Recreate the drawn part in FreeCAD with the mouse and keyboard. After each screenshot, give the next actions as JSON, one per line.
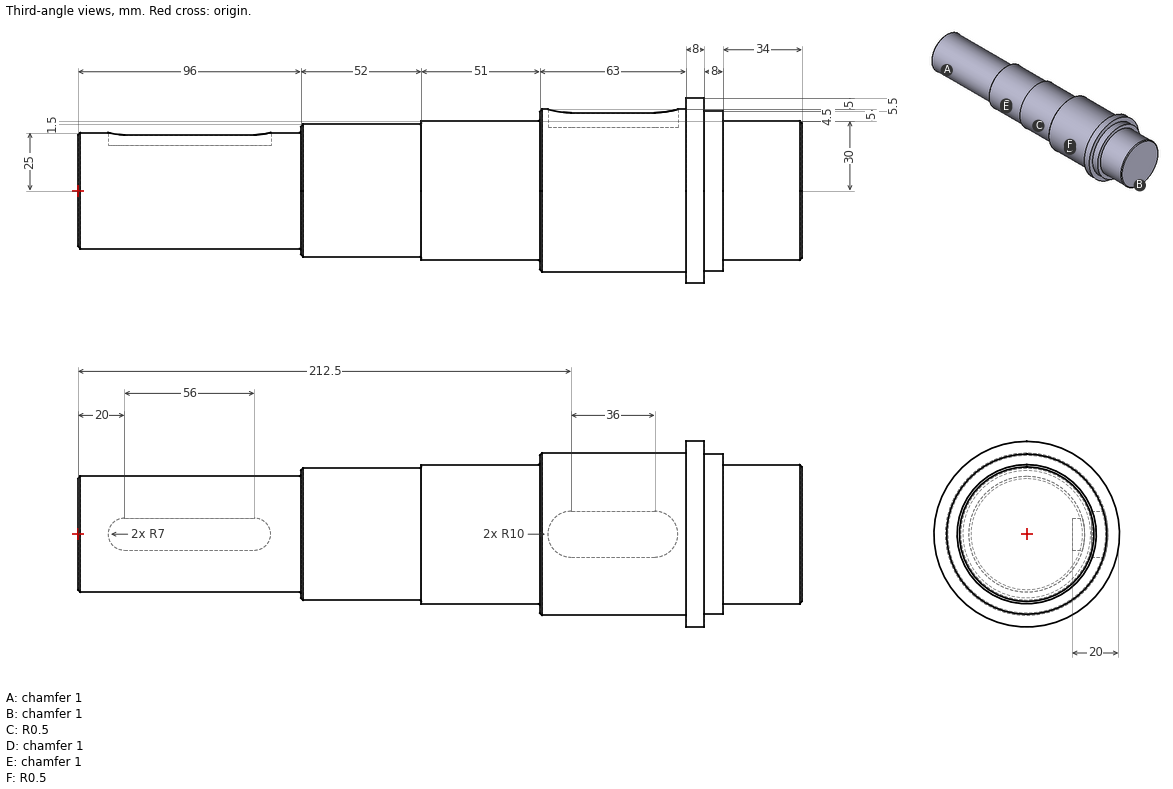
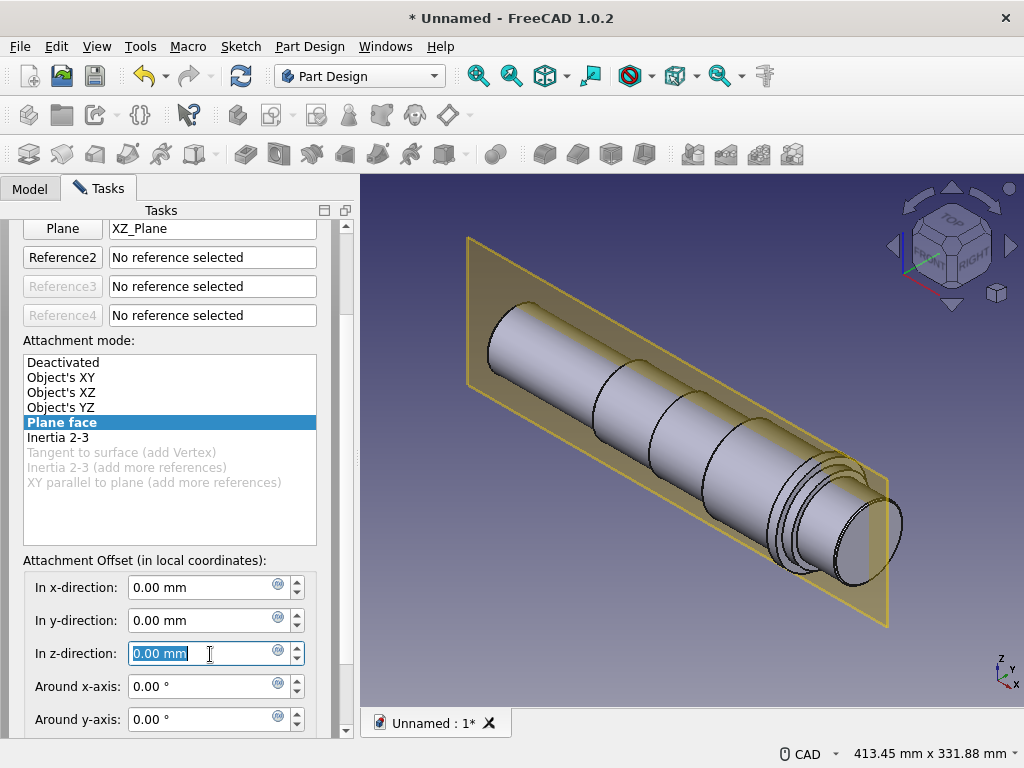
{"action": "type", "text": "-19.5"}
{"action": "key", "text": "Tab"}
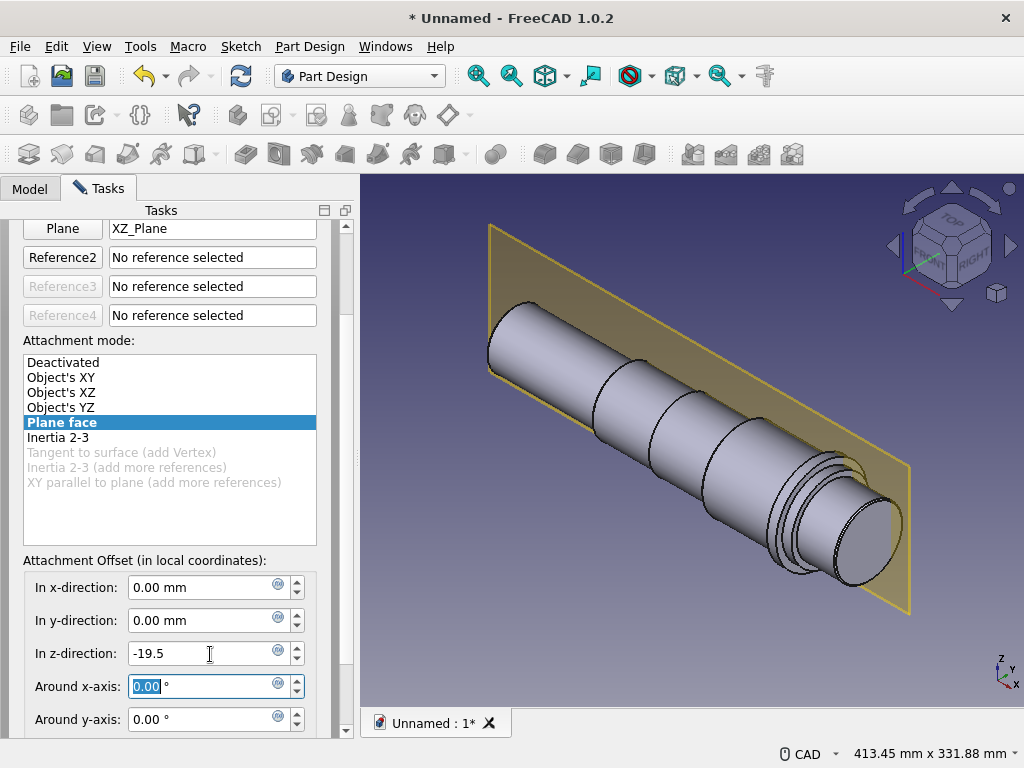
{"action": "scroll", "coordinate": [346, 479], "scroll_direction": "up", "scroll_amount": 3}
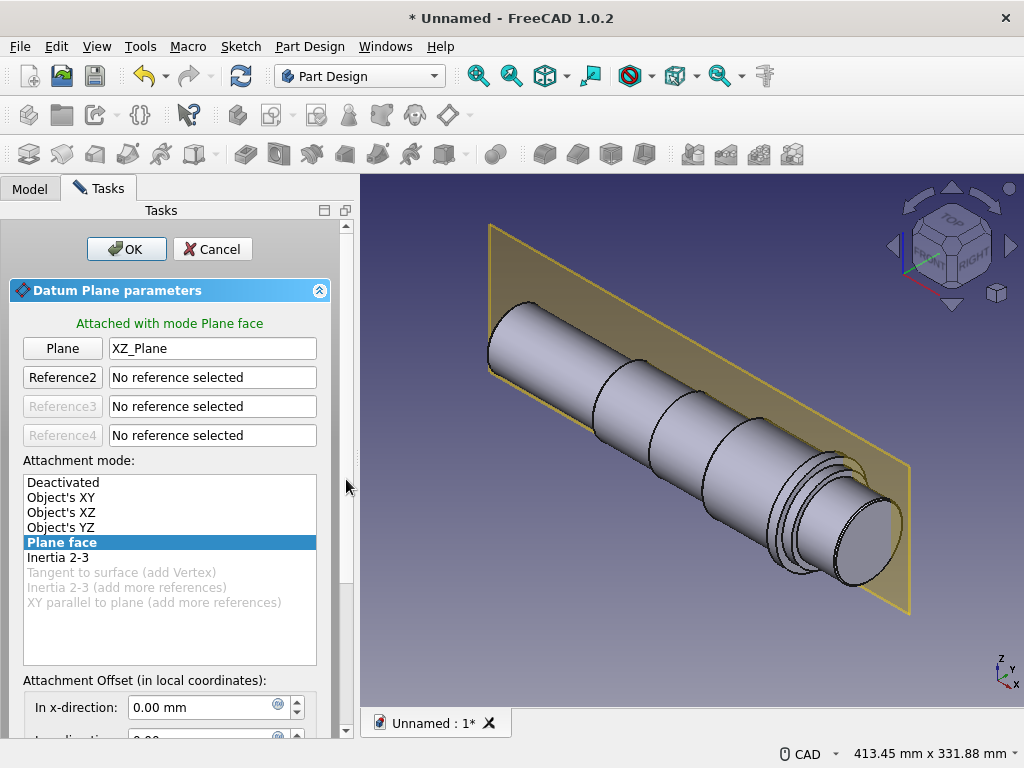
{"action": "left_click", "coordinate": [127, 249]}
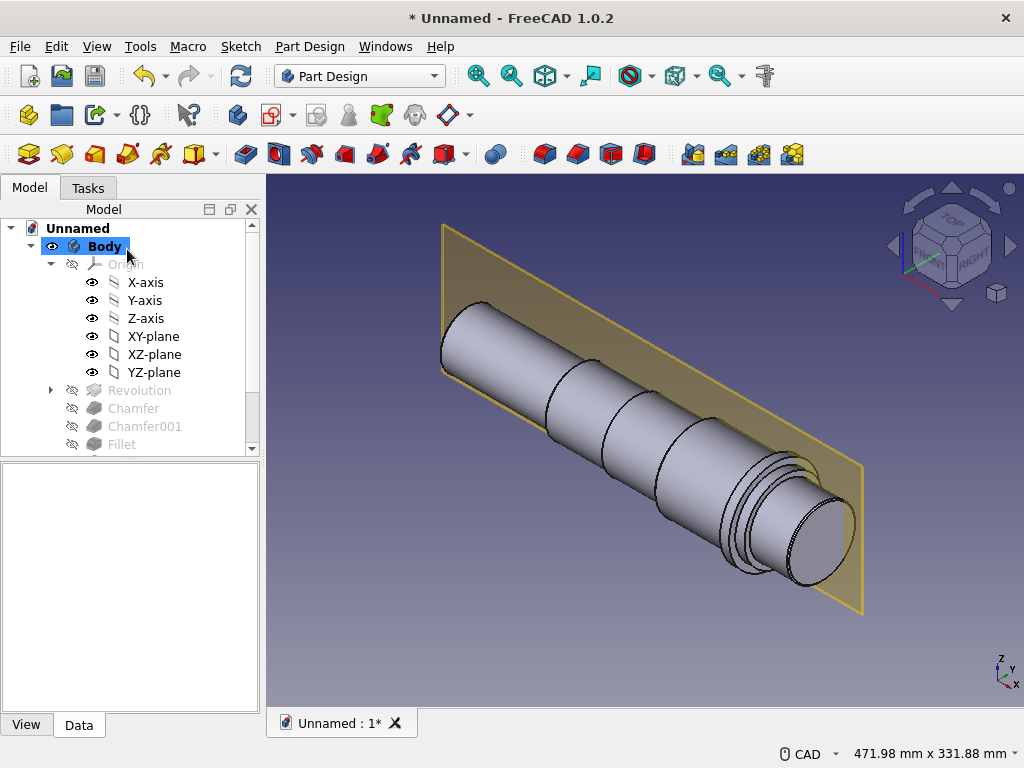
{"action": "scroll", "coordinate": [101, 332], "scroll_direction": "down", "scroll_amount": 3}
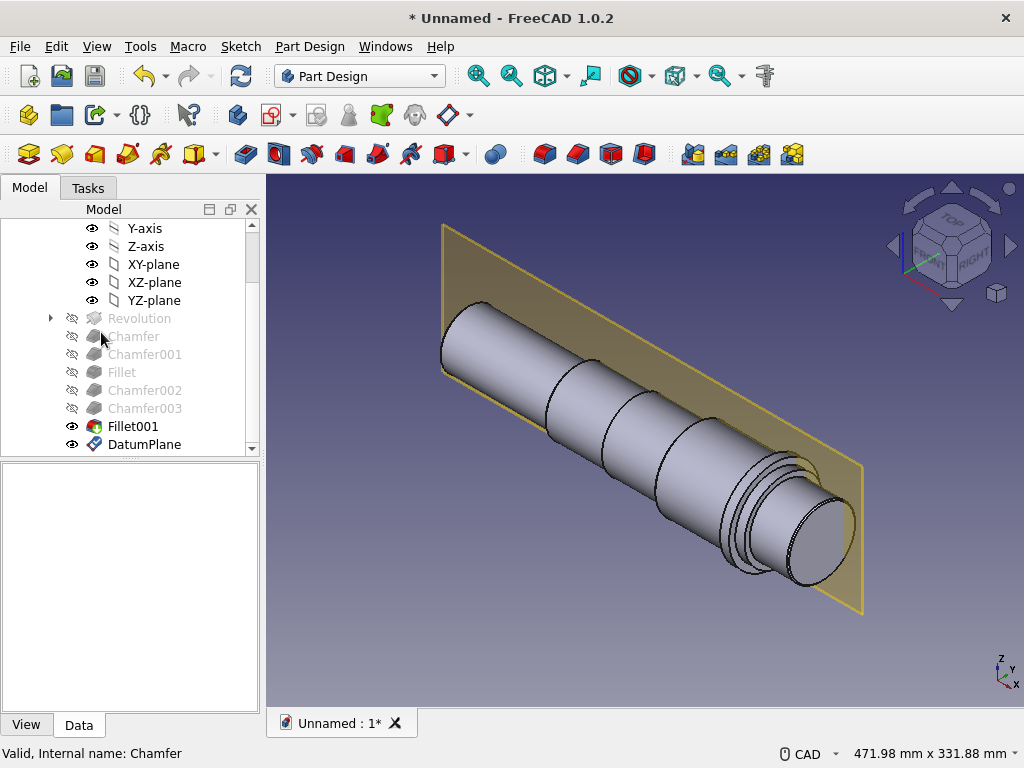
{"action": "left_click", "coordinate": [117, 444]}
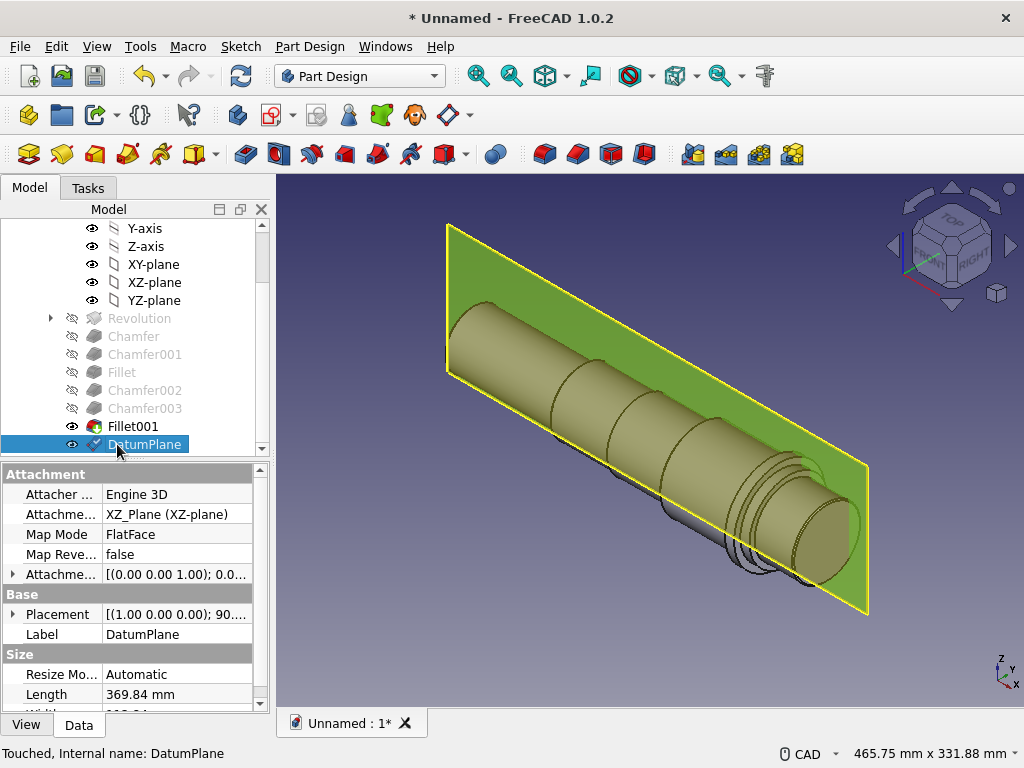
{"action": "left_click", "coordinate": [270, 116]}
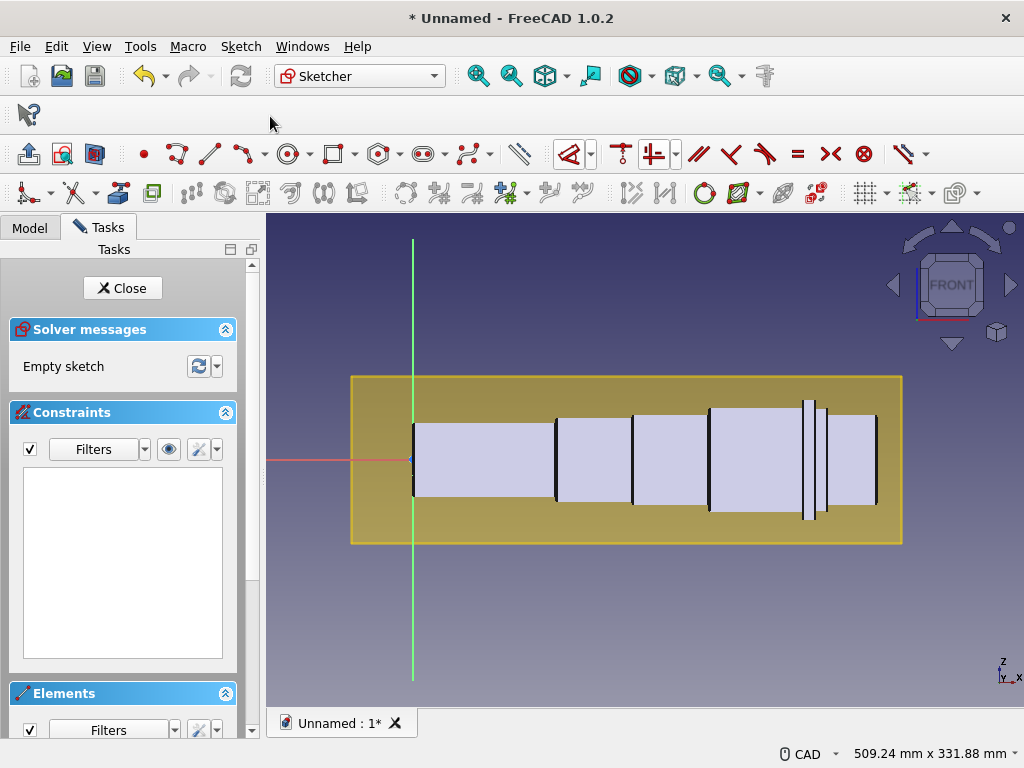
{"action": "left_click", "coordinate": [95, 154]}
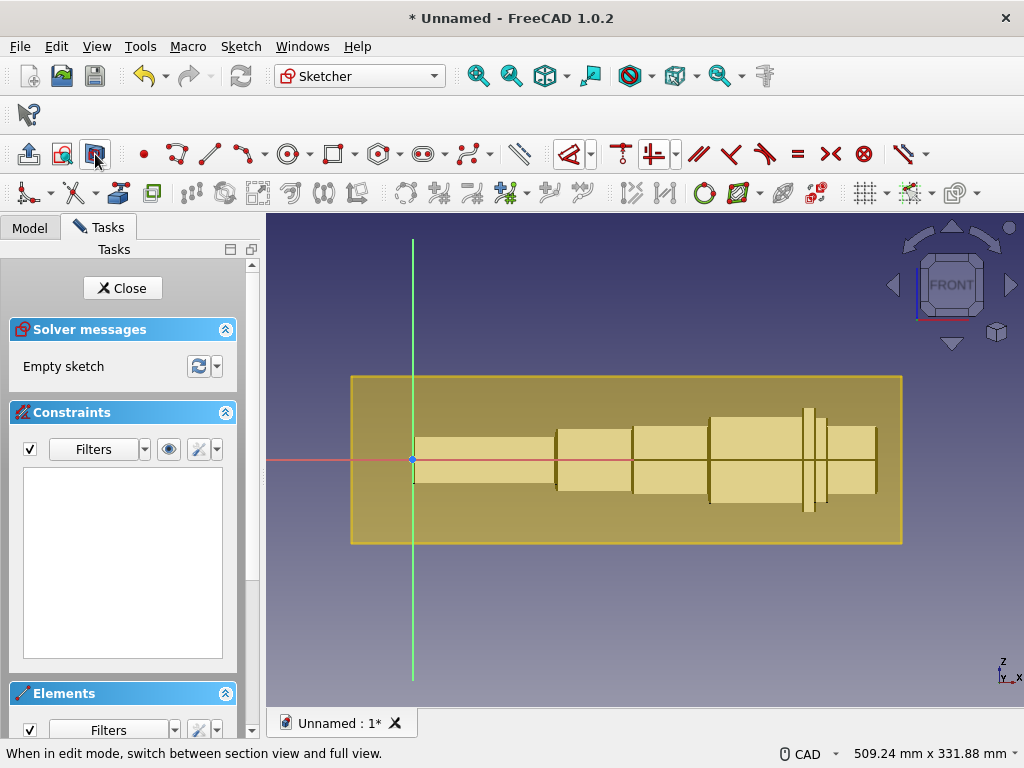
{"action": "scroll", "coordinate": [431, 460], "scroll_direction": "up", "scroll_amount": 6}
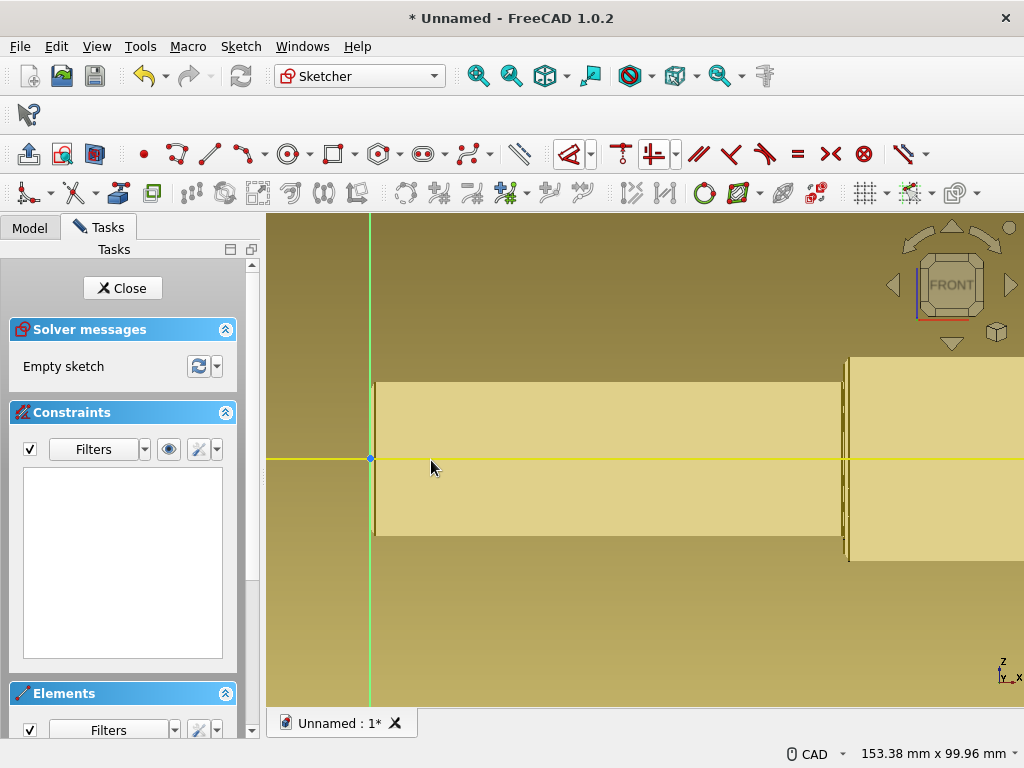
{"action": "key", "text": "g s"}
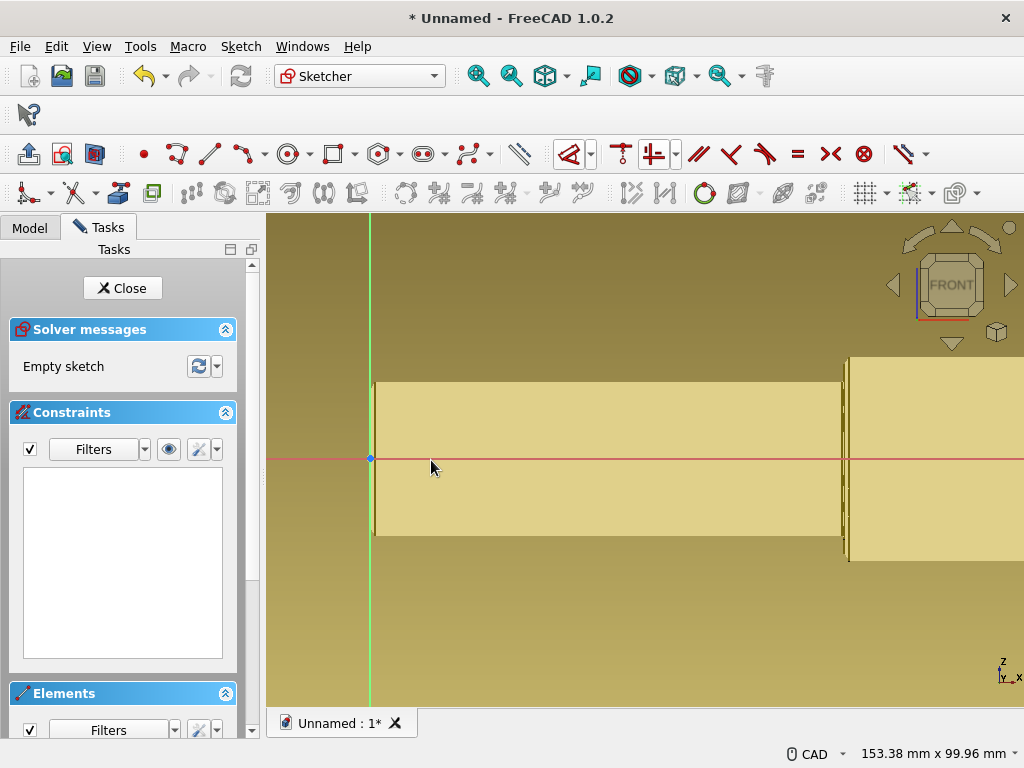
{"action": "left_click", "coordinate": [469, 459]}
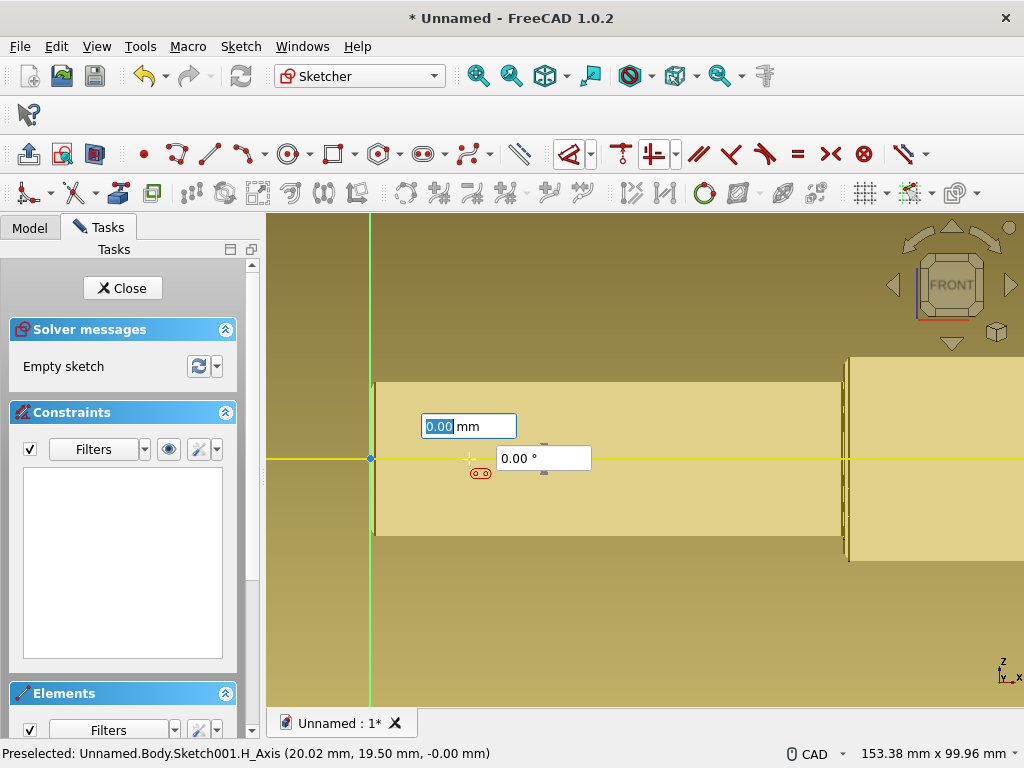
{"action": "left_click", "coordinate": [746, 450]}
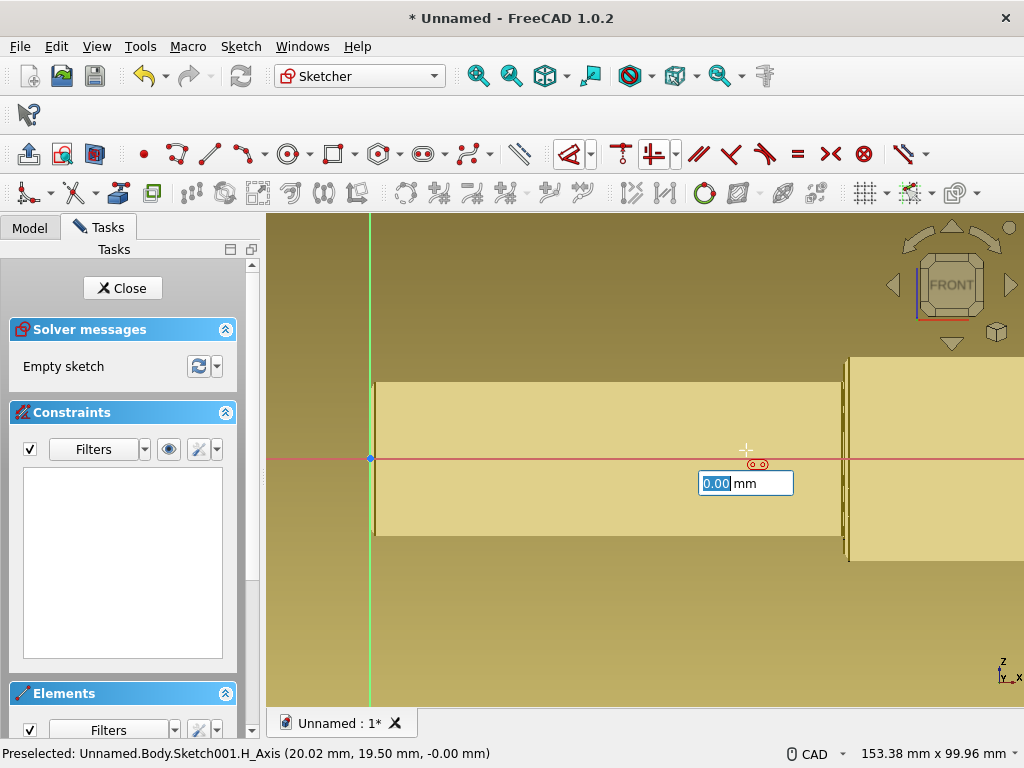
{"action": "left_click", "coordinate": [607, 493]}
{"action": "key", "text": "Escape"}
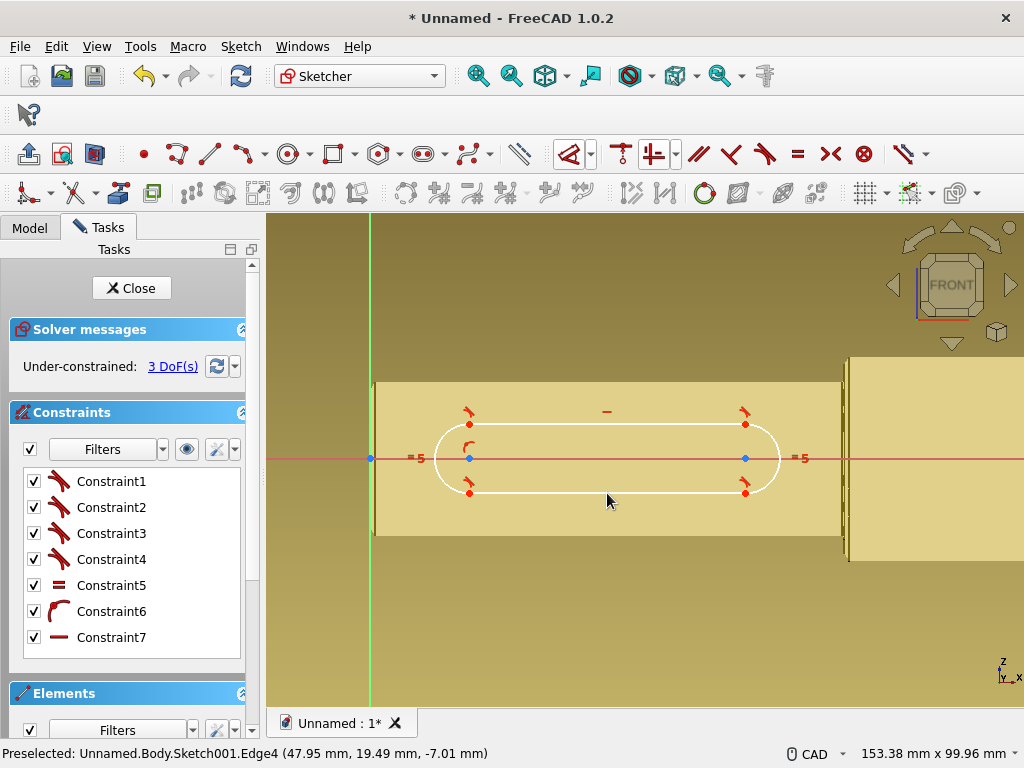
{"action": "left_click", "coordinate": [442, 438]}